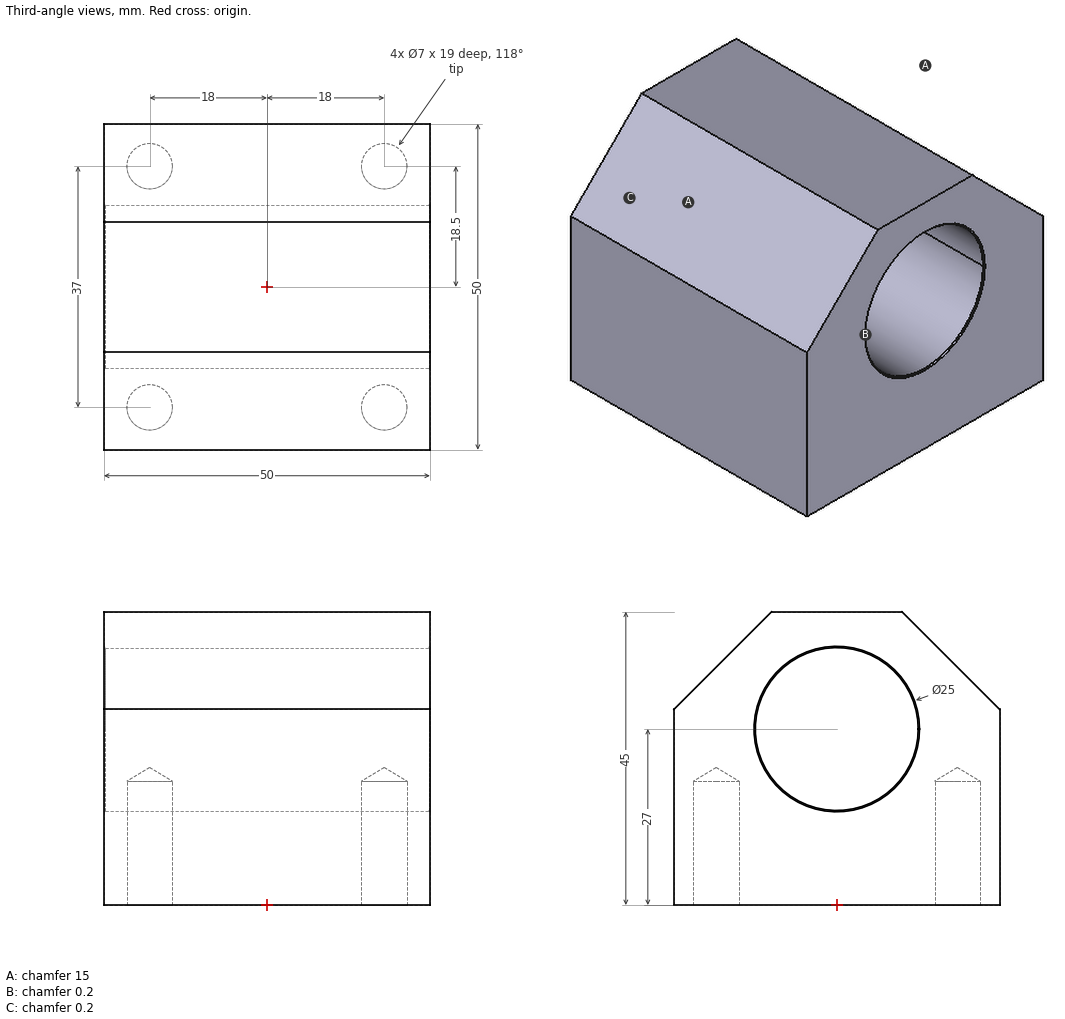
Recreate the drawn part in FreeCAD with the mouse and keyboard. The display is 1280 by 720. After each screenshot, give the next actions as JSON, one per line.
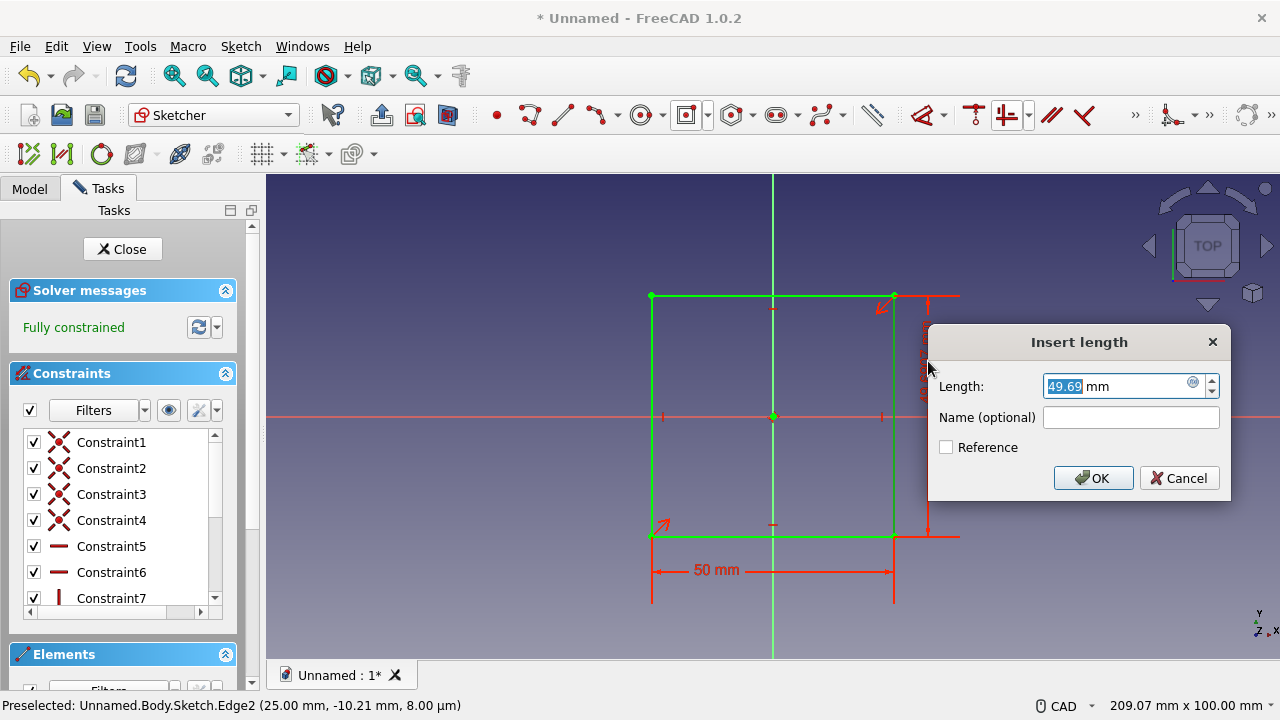
{"action": "type", "text": "50"}
{"action": "key", "text": "Return"}
{"action": "key", "text": "Escape"}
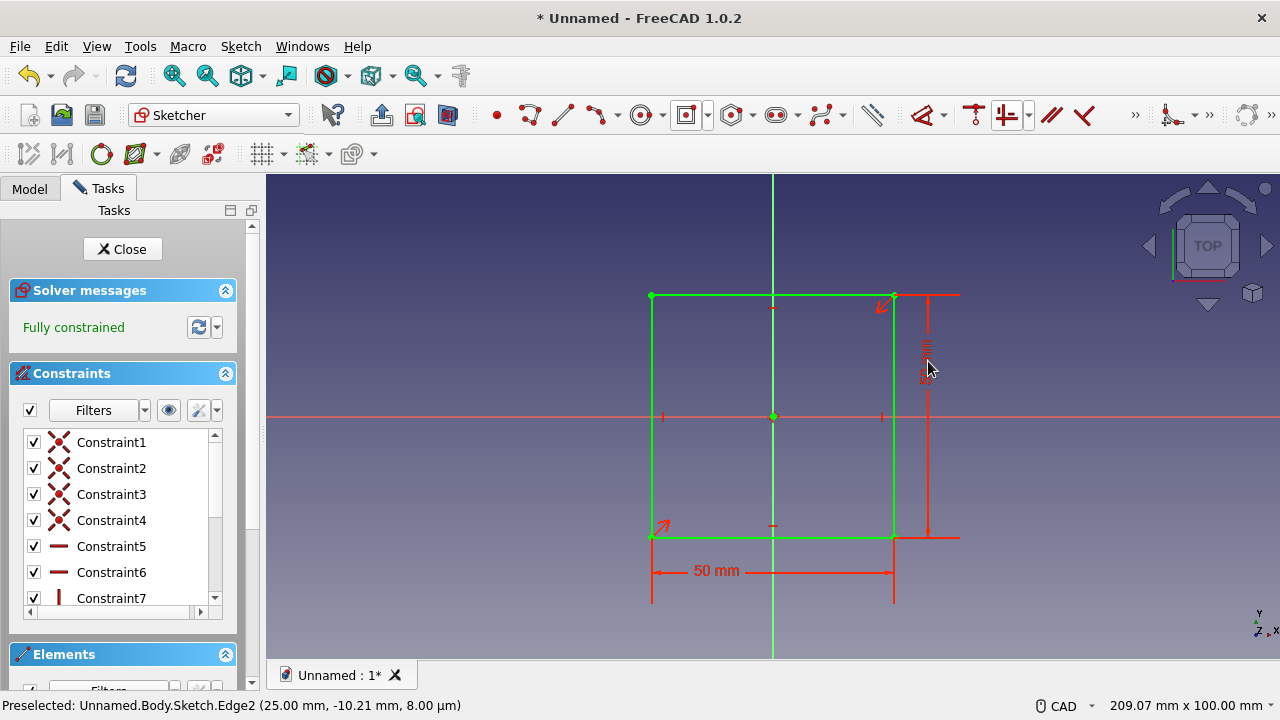
{"action": "left_click", "coordinate": [123, 249]}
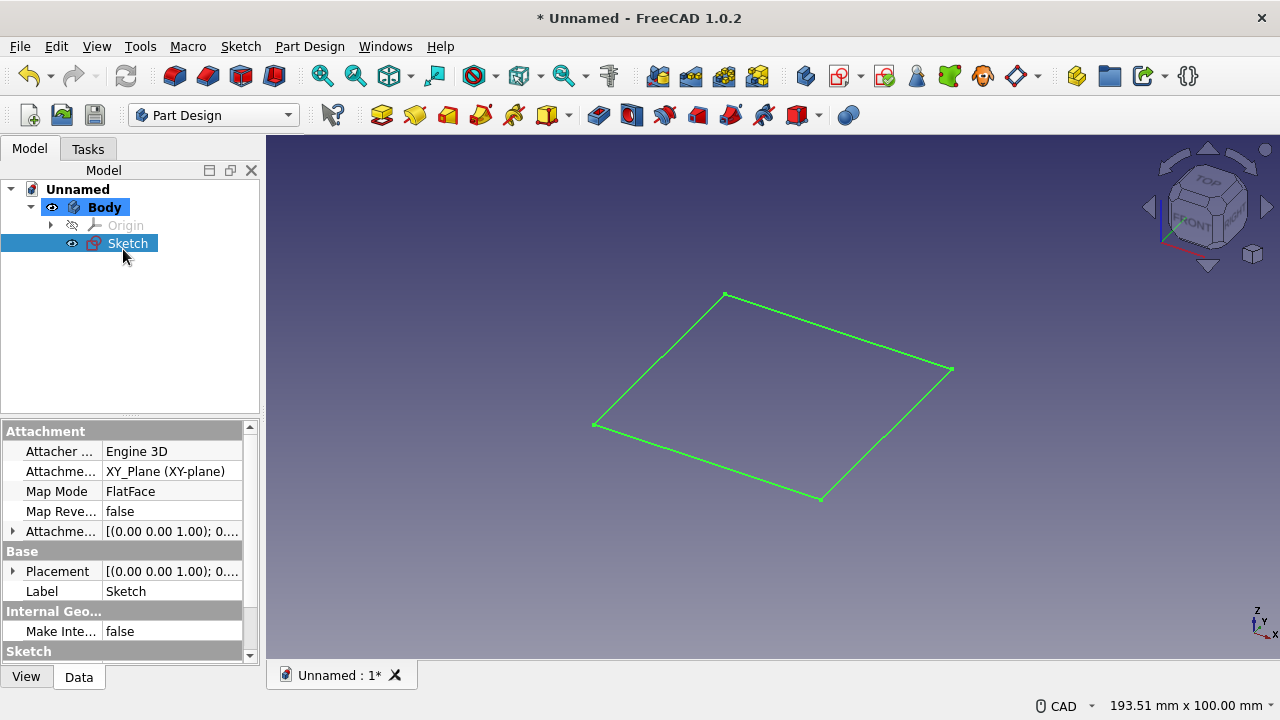
{"action": "left_click", "coordinate": [382, 116]}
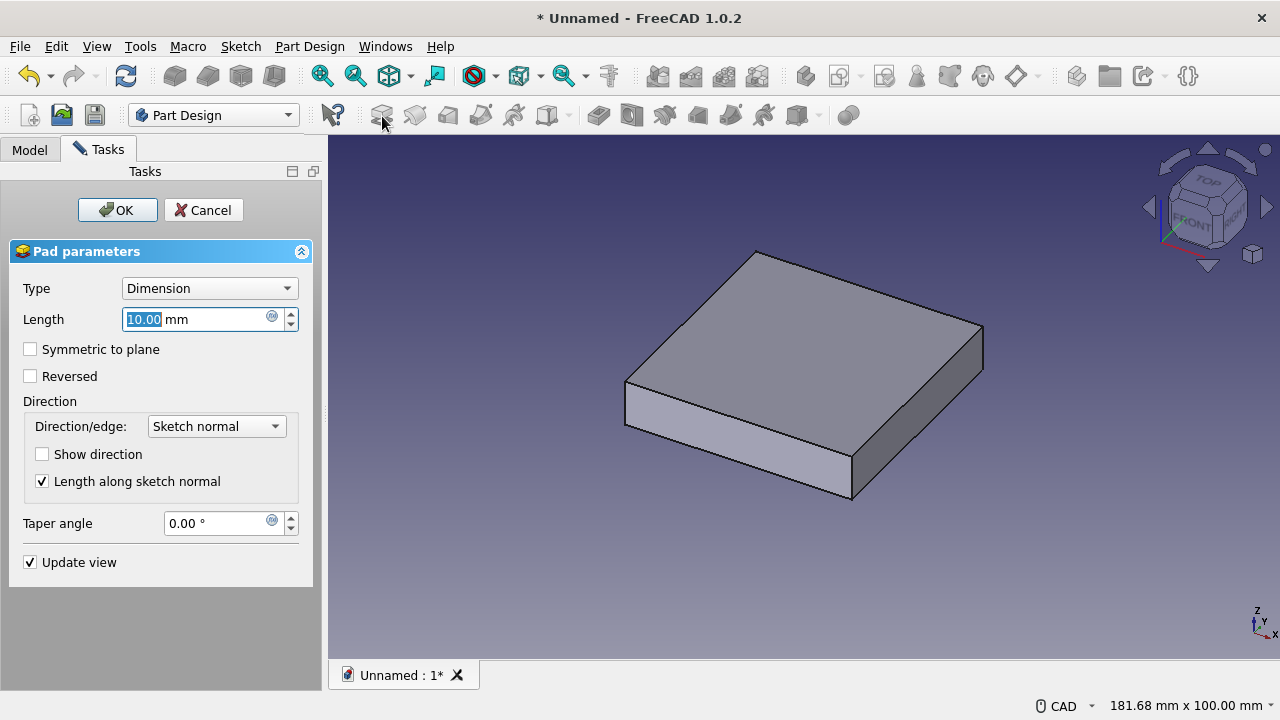
{"action": "type", "text": "45"}
{"action": "key", "text": "Tab"}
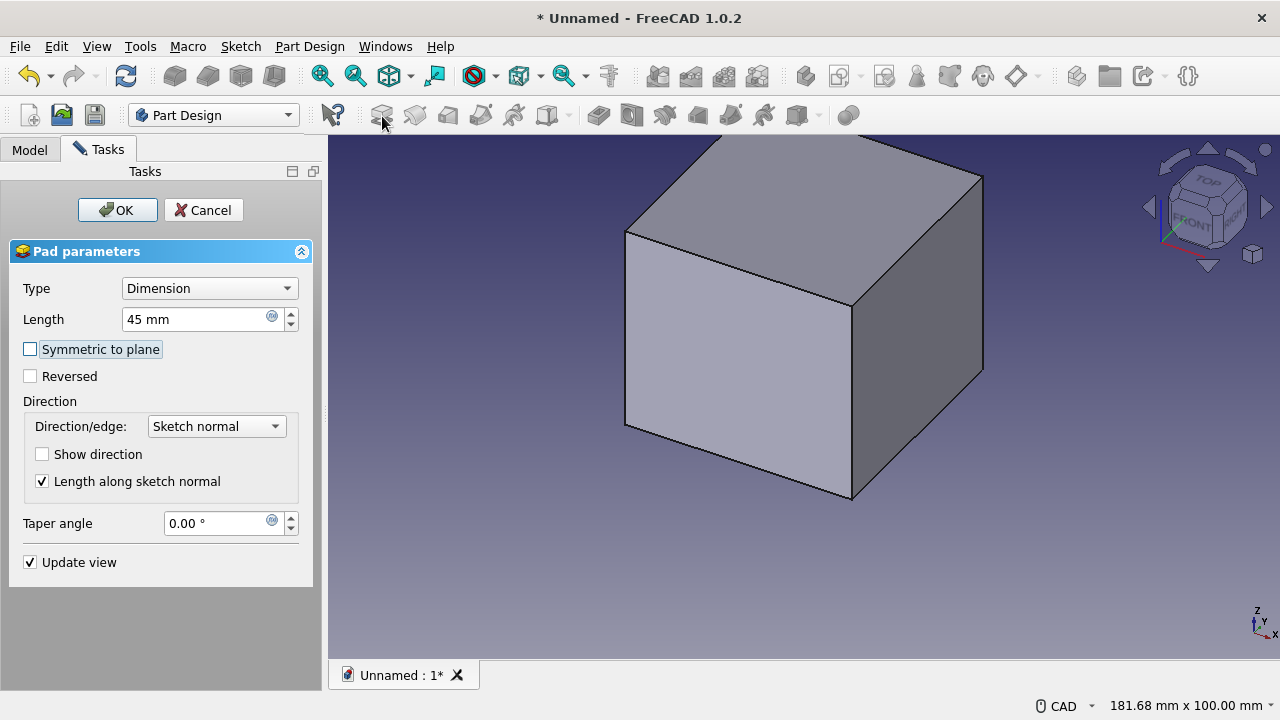
{"action": "left_click", "coordinate": [118, 210]}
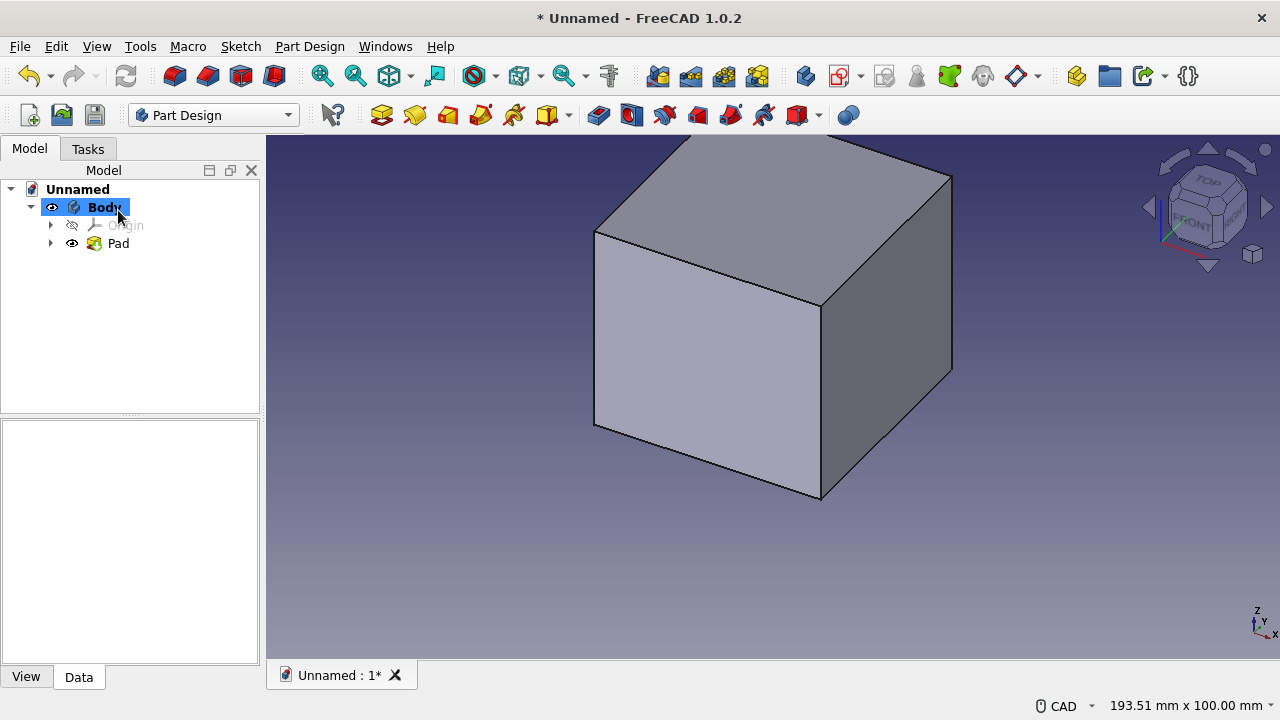
{"action": "left_click", "coordinate": [323, 76]}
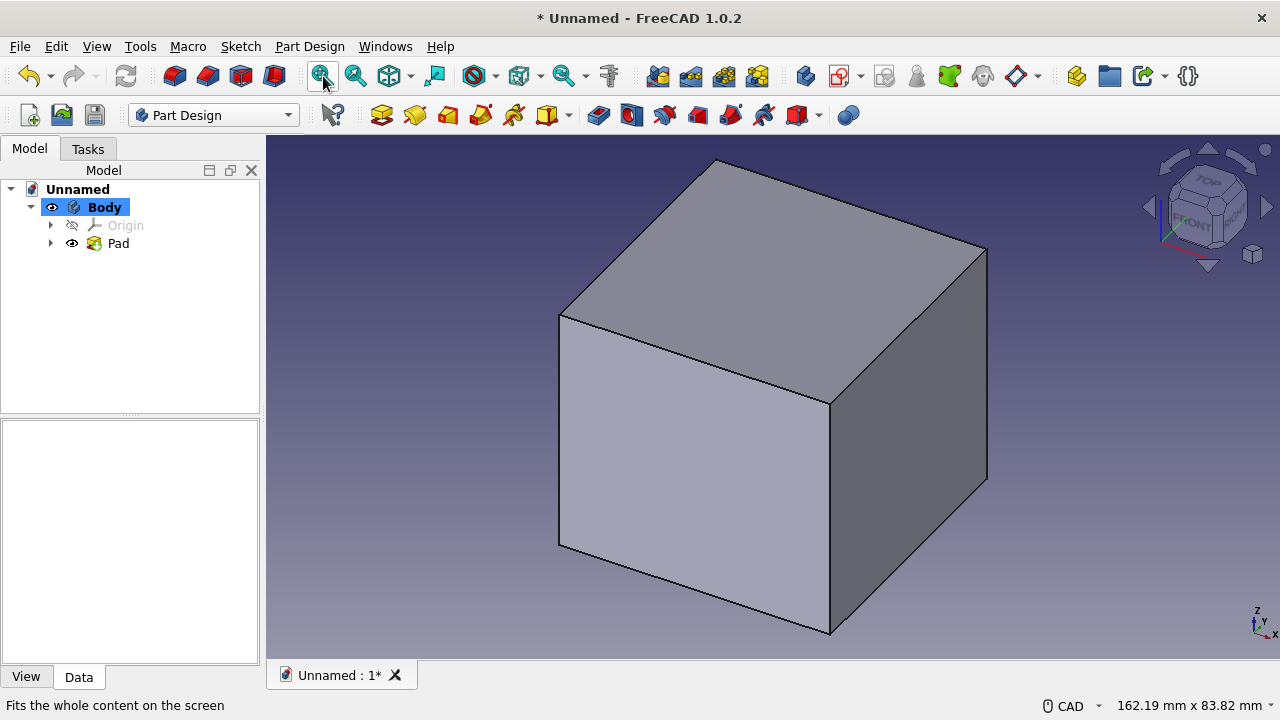
{"action": "left_click", "coordinate": [908, 441]}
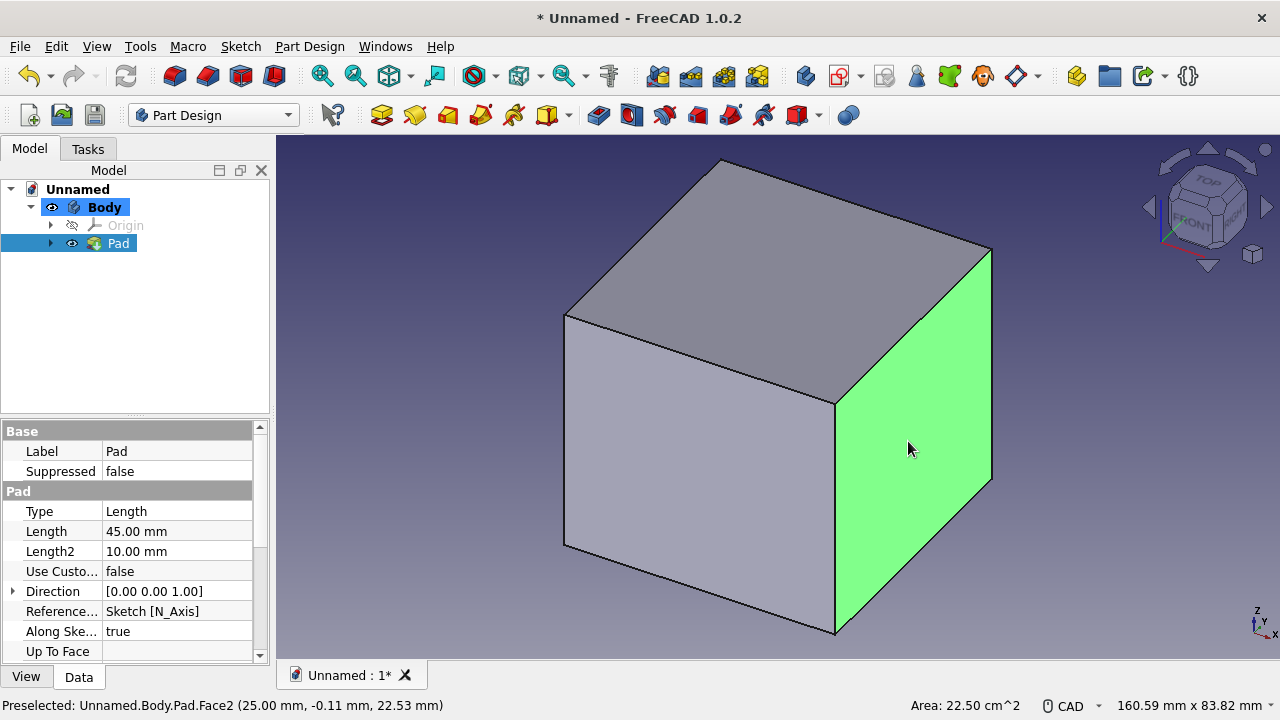
{"action": "left_click", "coordinate": [838, 76]}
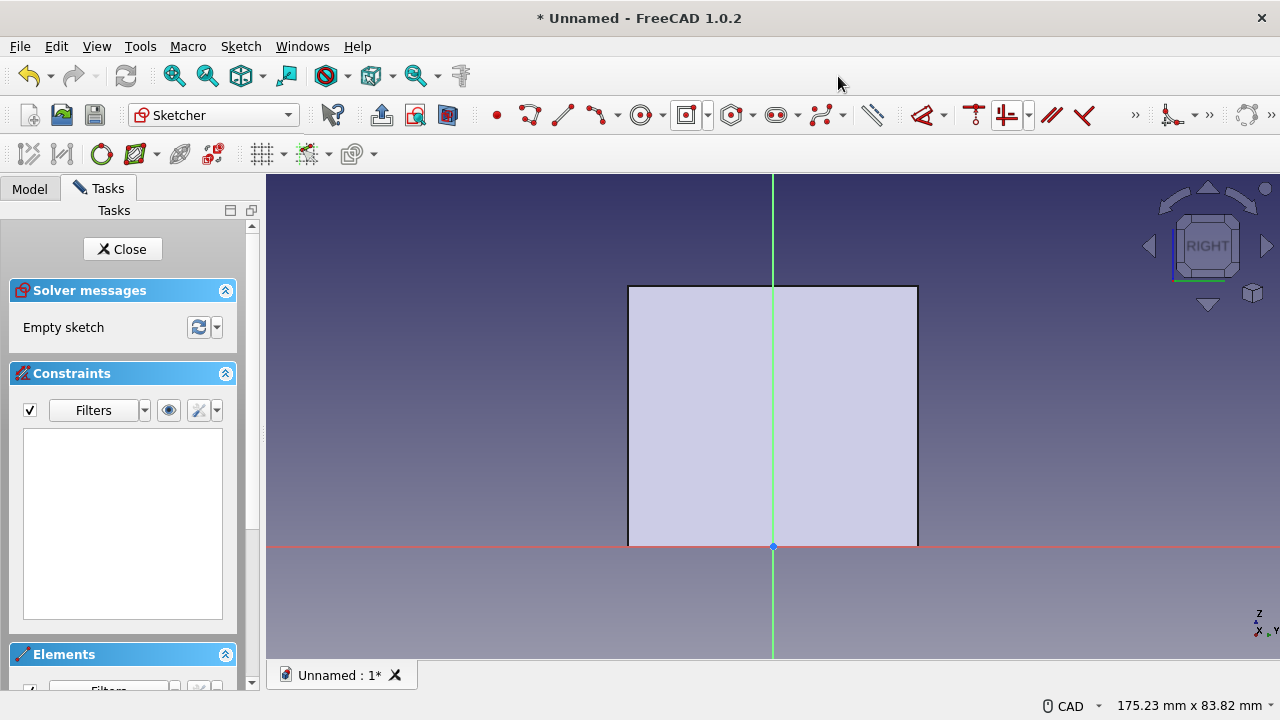
{"action": "left_click", "coordinate": [640, 116]}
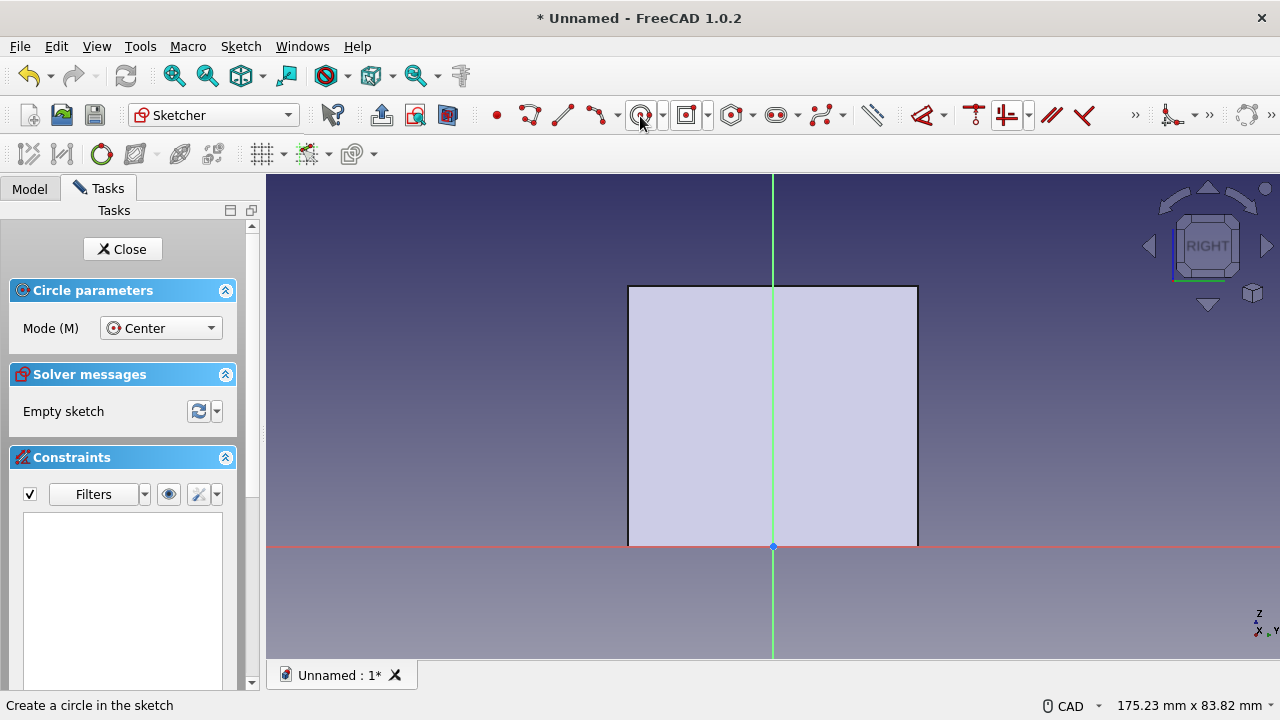
{"action": "left_click", "coordinate": [773, 390]}
{"action": "left_click", "coordinate": [824, 339]}
{"action": "key", "text": "Escape"}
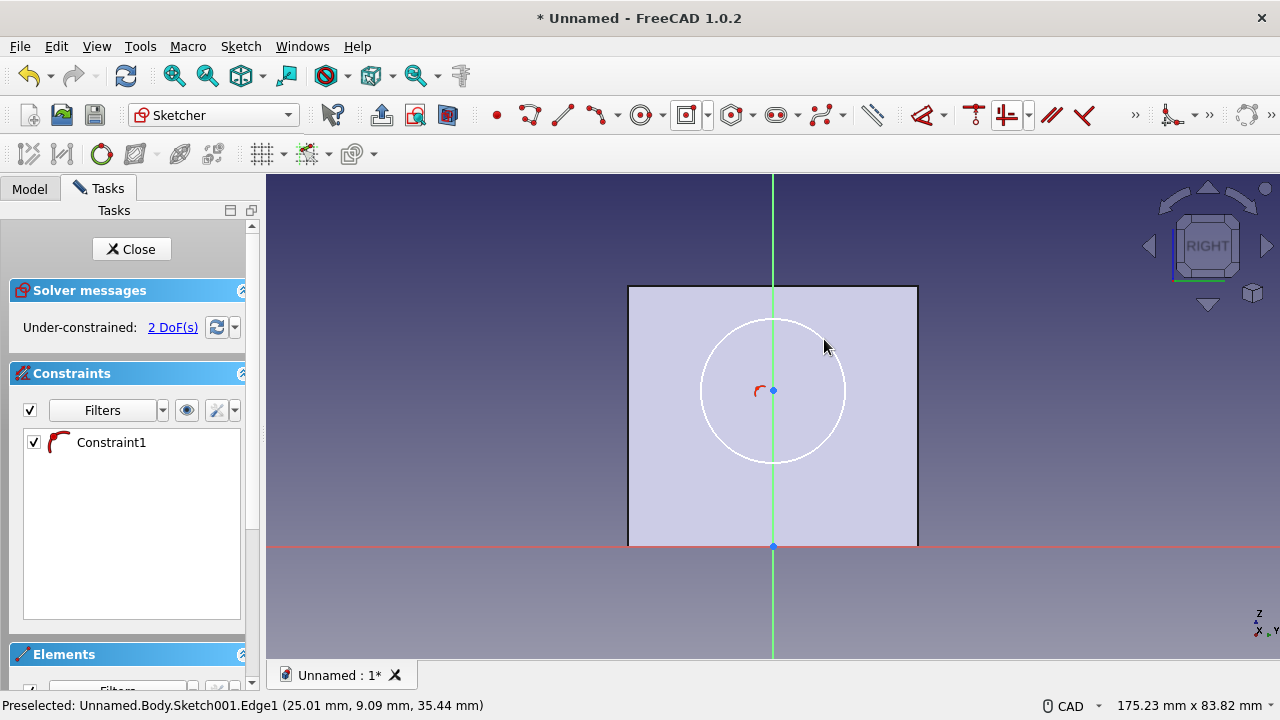
{"action": "left_click", "coordinate": [922, 116]}